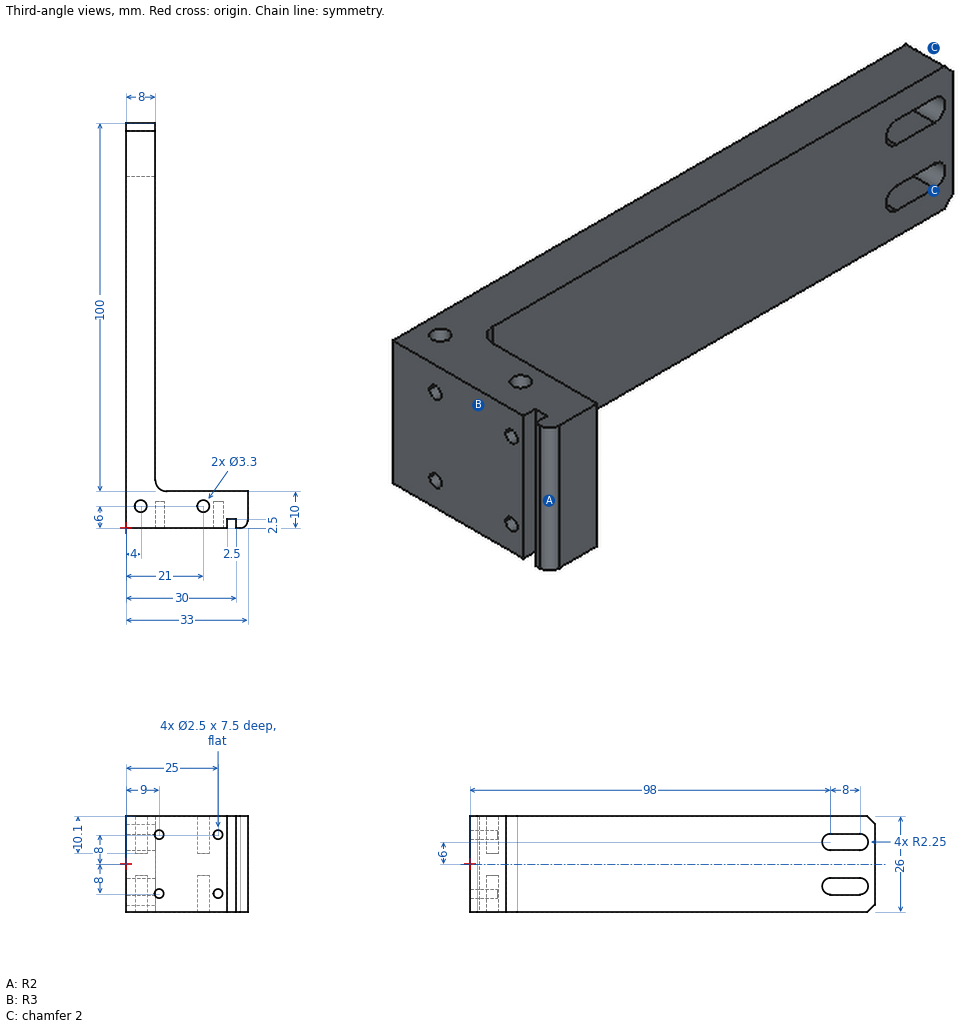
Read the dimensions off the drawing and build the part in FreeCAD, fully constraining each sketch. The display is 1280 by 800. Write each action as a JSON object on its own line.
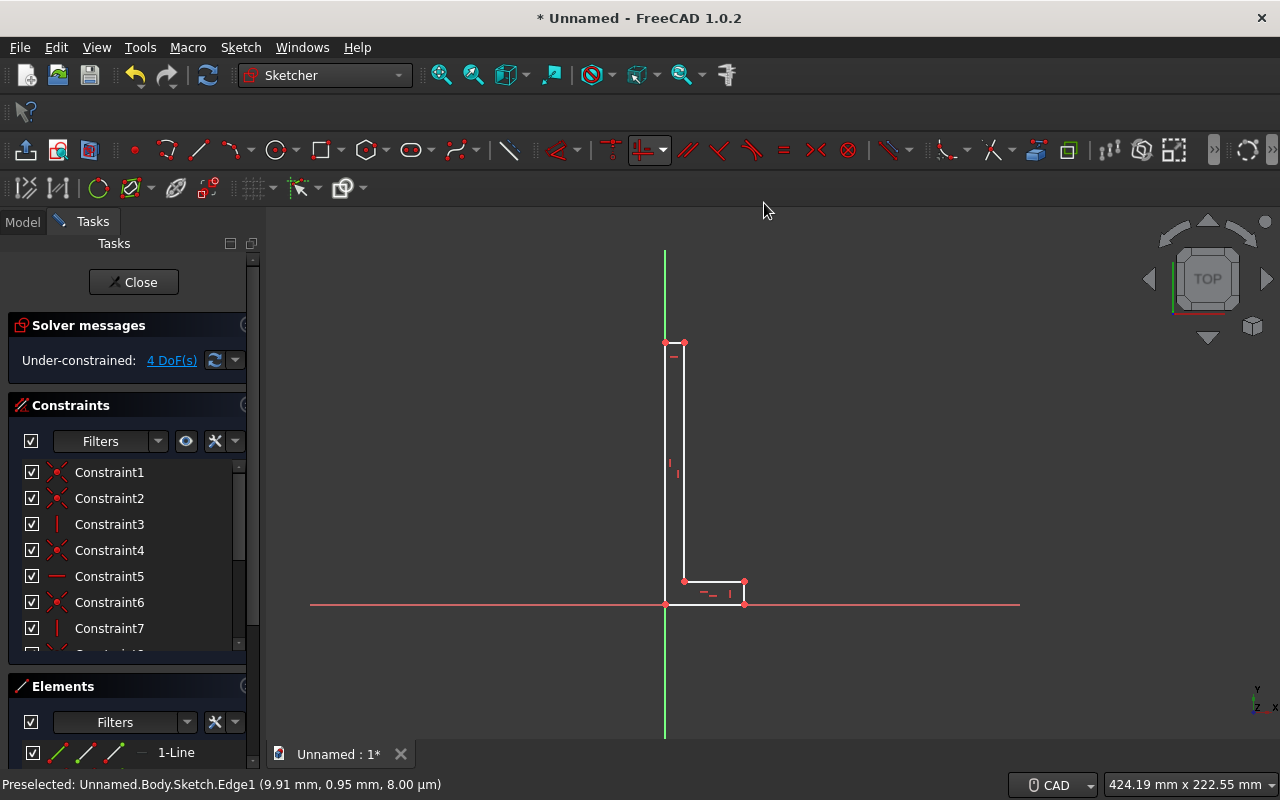
{"action": "left_click", "coordinate": [556, 150]}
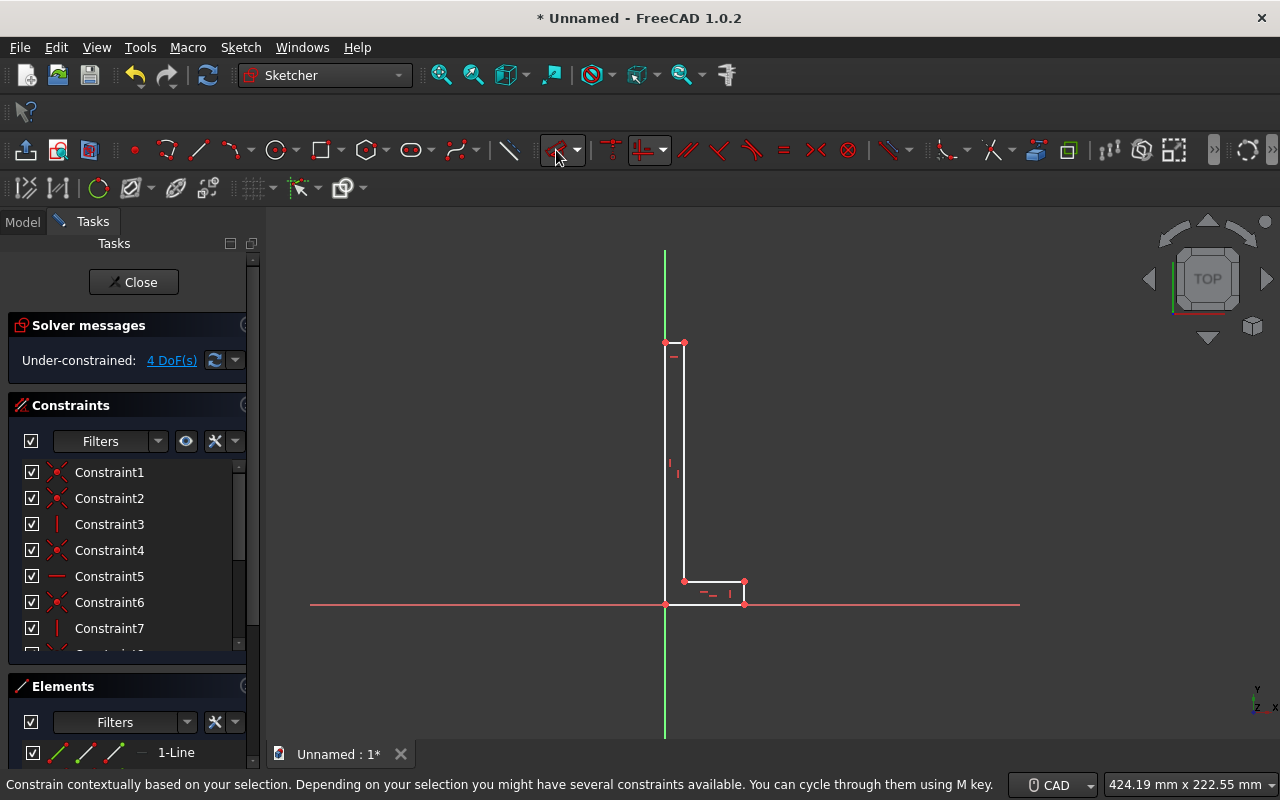
{"action": "scroll", "coordinate": [675, 343], "scroll_direction": "up", "scroll_amount": 4}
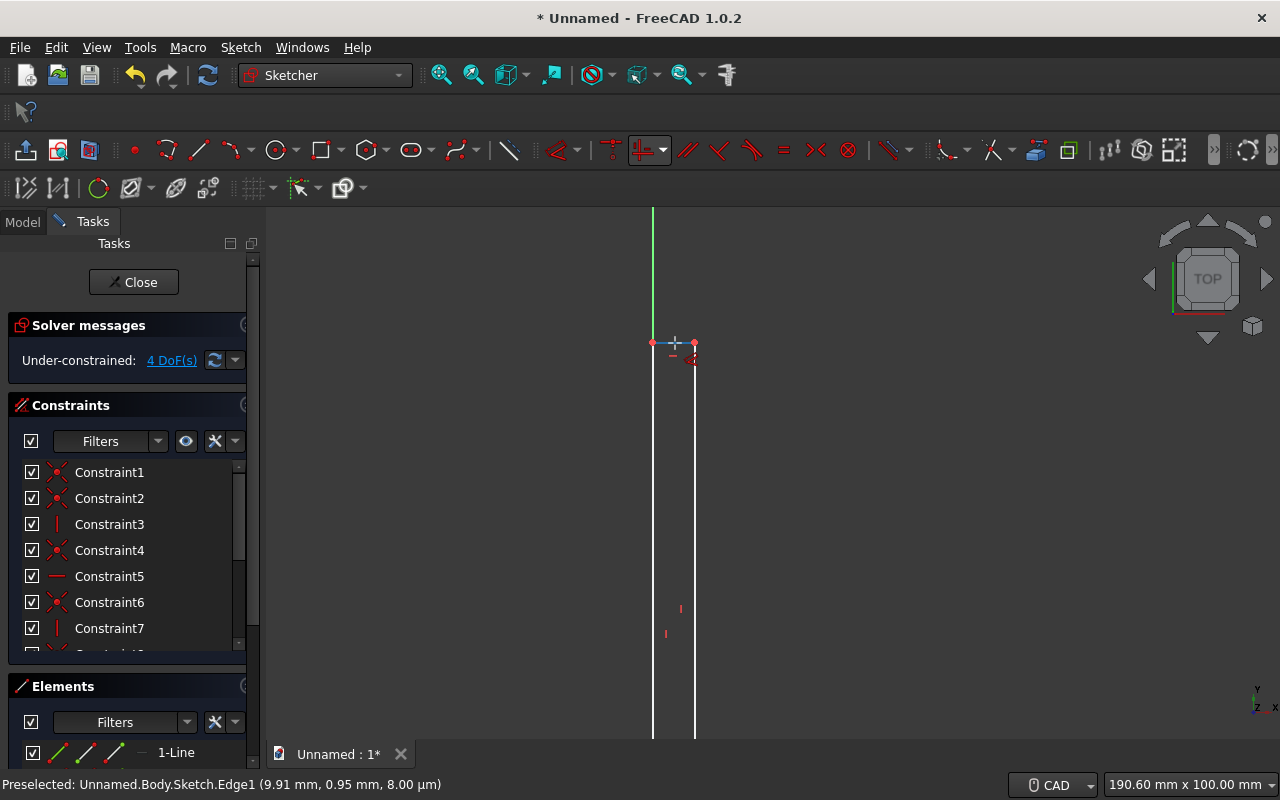
{"action": "left_click", "coordinate": [674, 343]}
{"action": "left_click", "coordinate": [674, 309]}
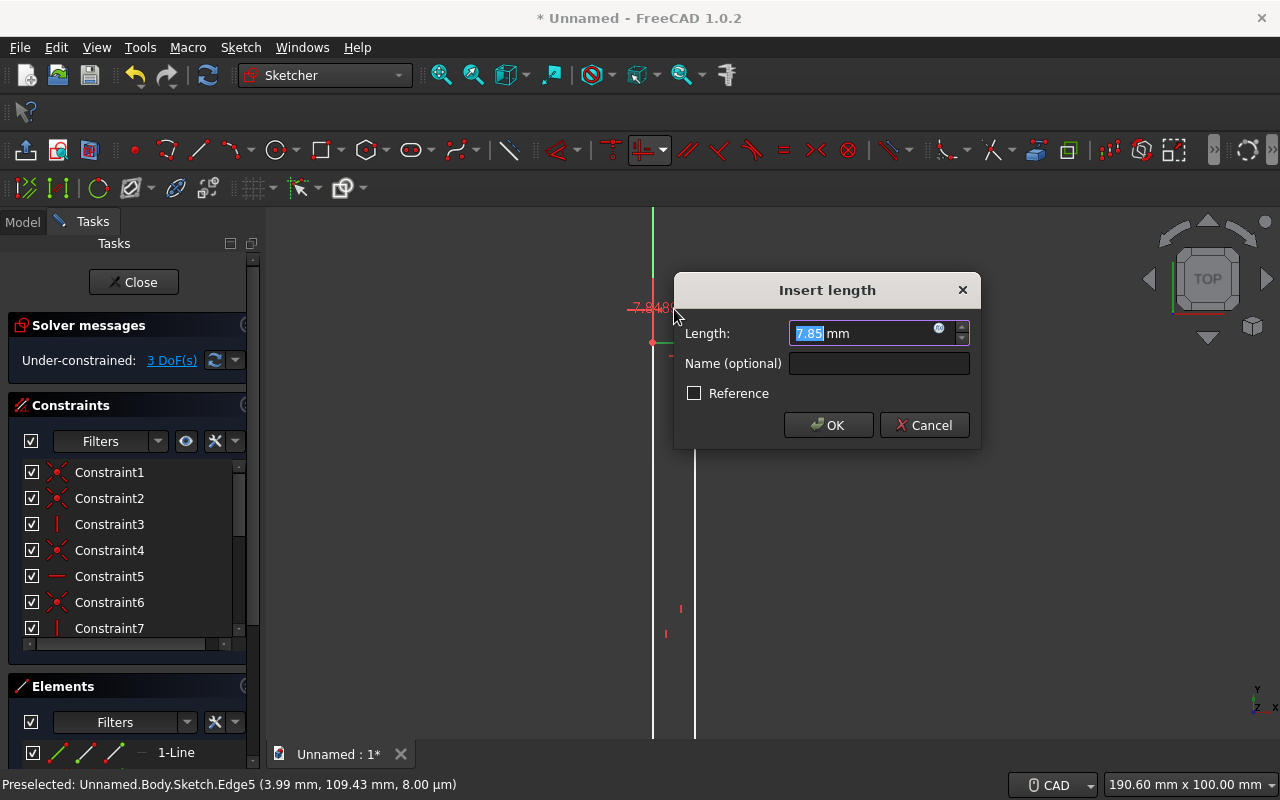
{"action": "type", "text": "8"}
{"action": "key", "text": "Return"}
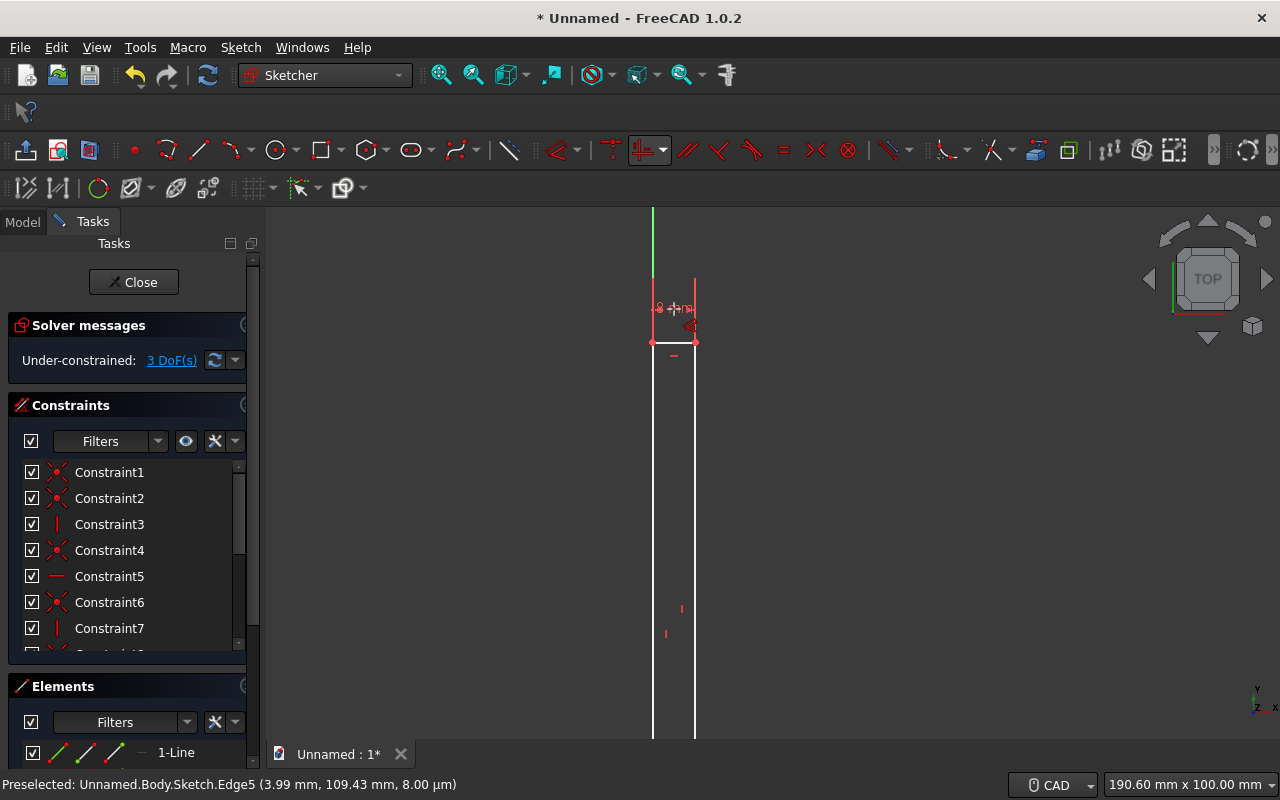
{"action": "scroll", "coordinate": [661, 279], "scroll_direction": "down", "scroll_amount": 3}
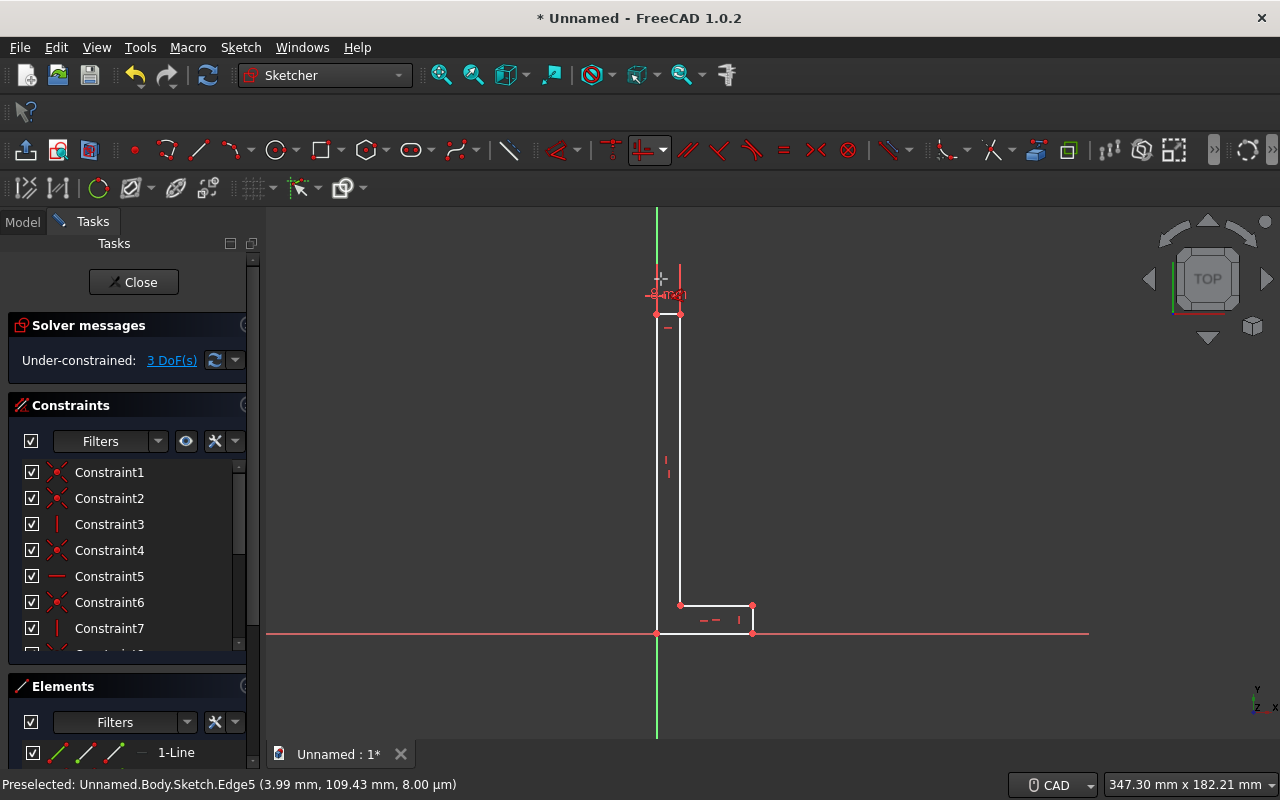
{"action": "left_click", "coordinate": [686, 634]}
{"action": "left_click", "coordinate": [705, 668]}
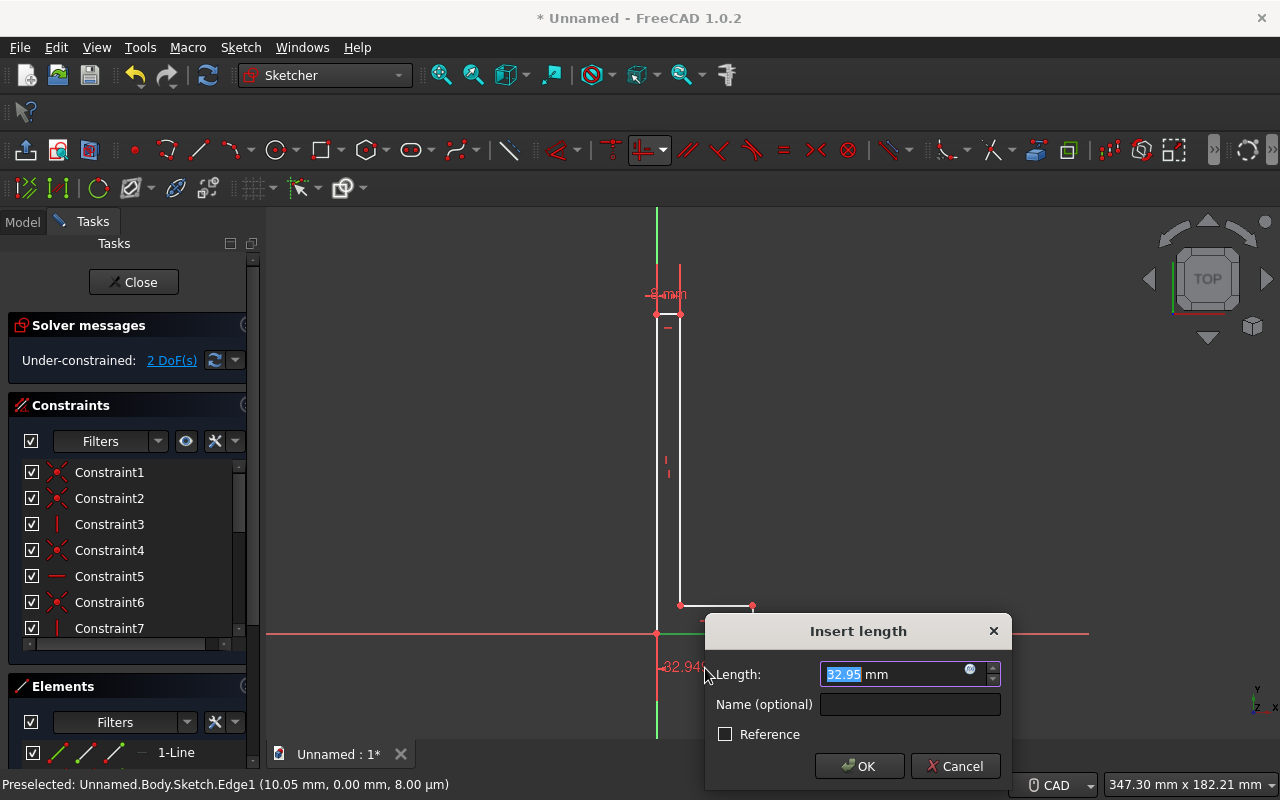
{"action": "type", "text": "33"}
{"action": "key", "text": "Return"}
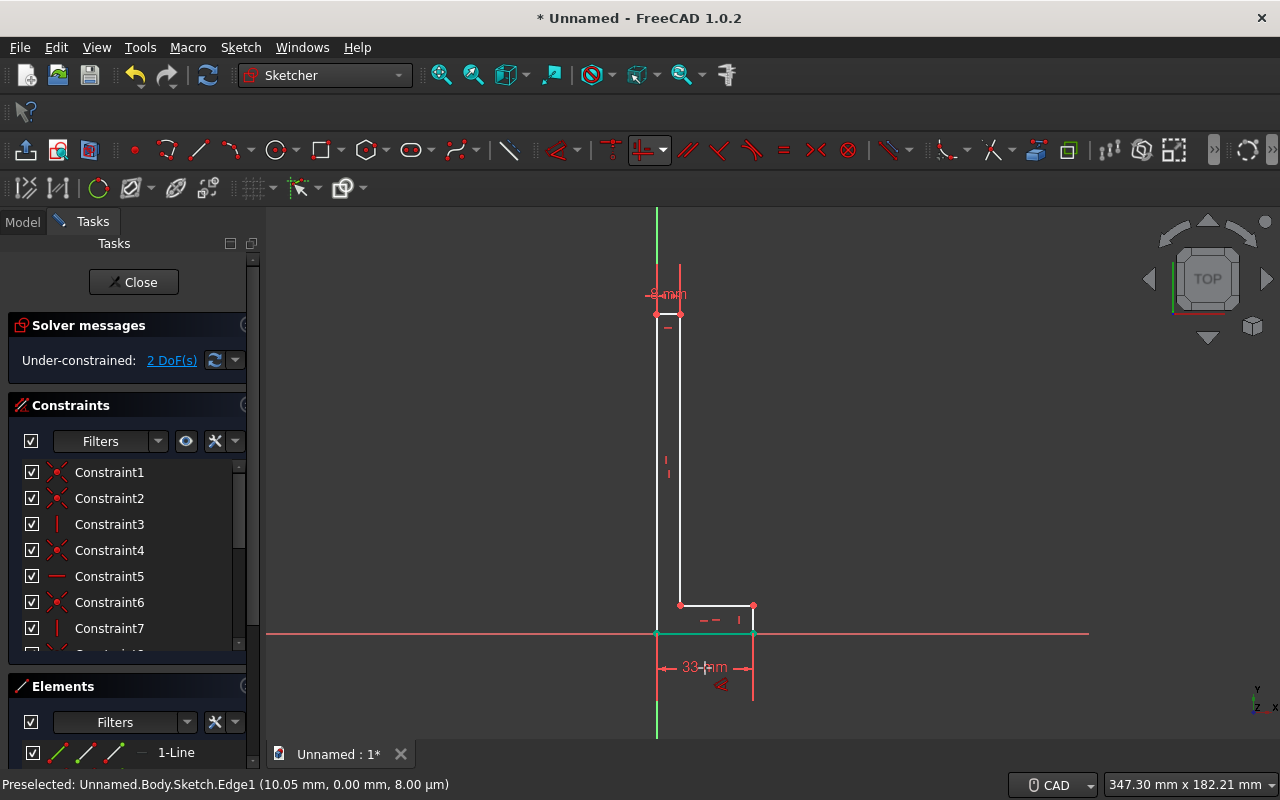
{"action": "scroll", "coordinate": [753, 622], "scroll_direction": "up", "scroll_amount": 2}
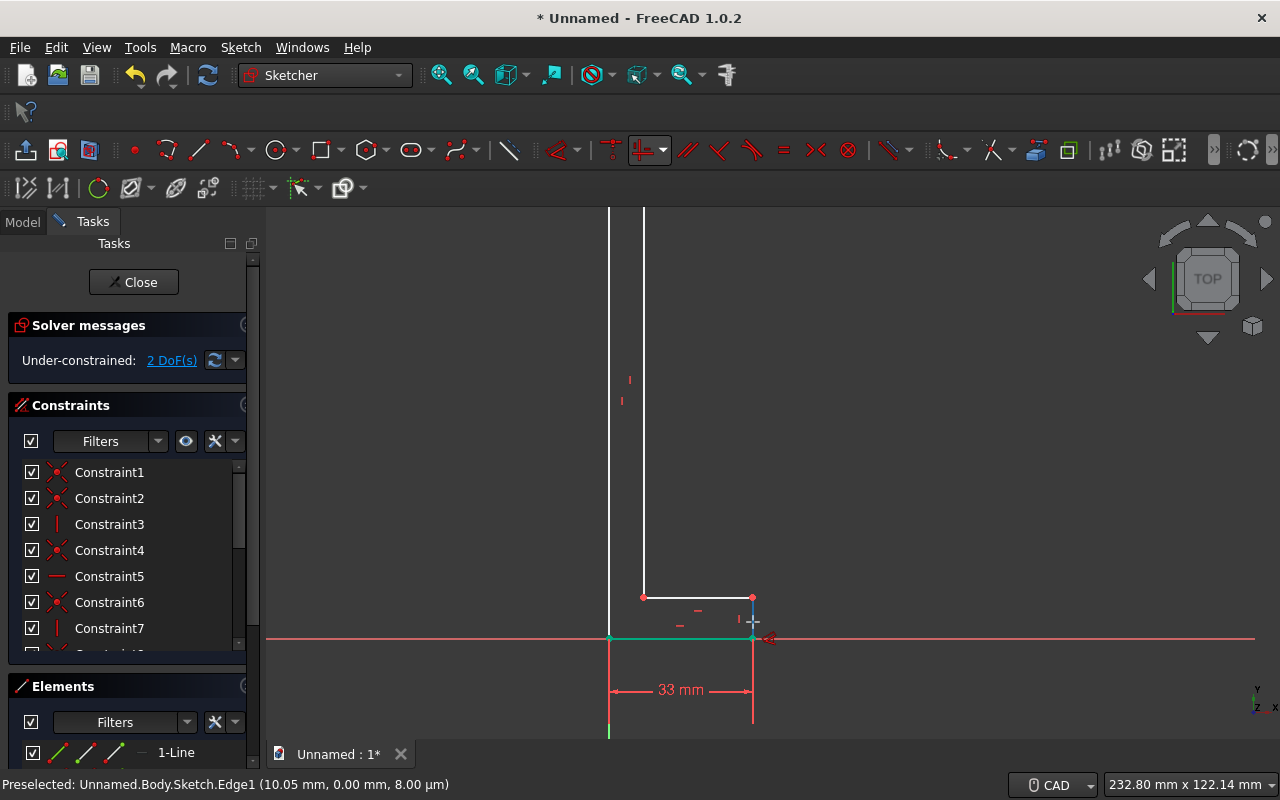
{"action": "left_click", "coordinate": [753, 622]}
{"action": "left_click", "coordinate": [787, 618]}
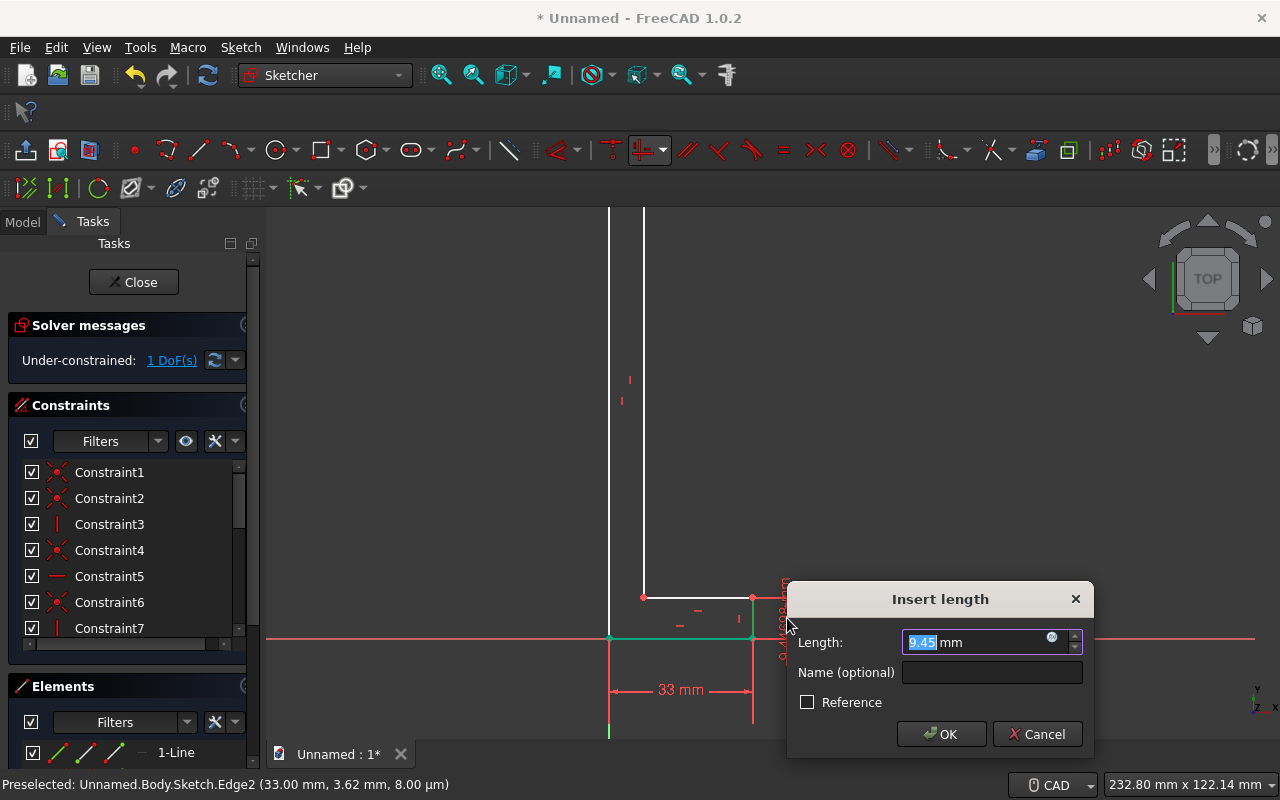
{"action": "type", "text": "10"}
{"action": "key", "text": "Return"}